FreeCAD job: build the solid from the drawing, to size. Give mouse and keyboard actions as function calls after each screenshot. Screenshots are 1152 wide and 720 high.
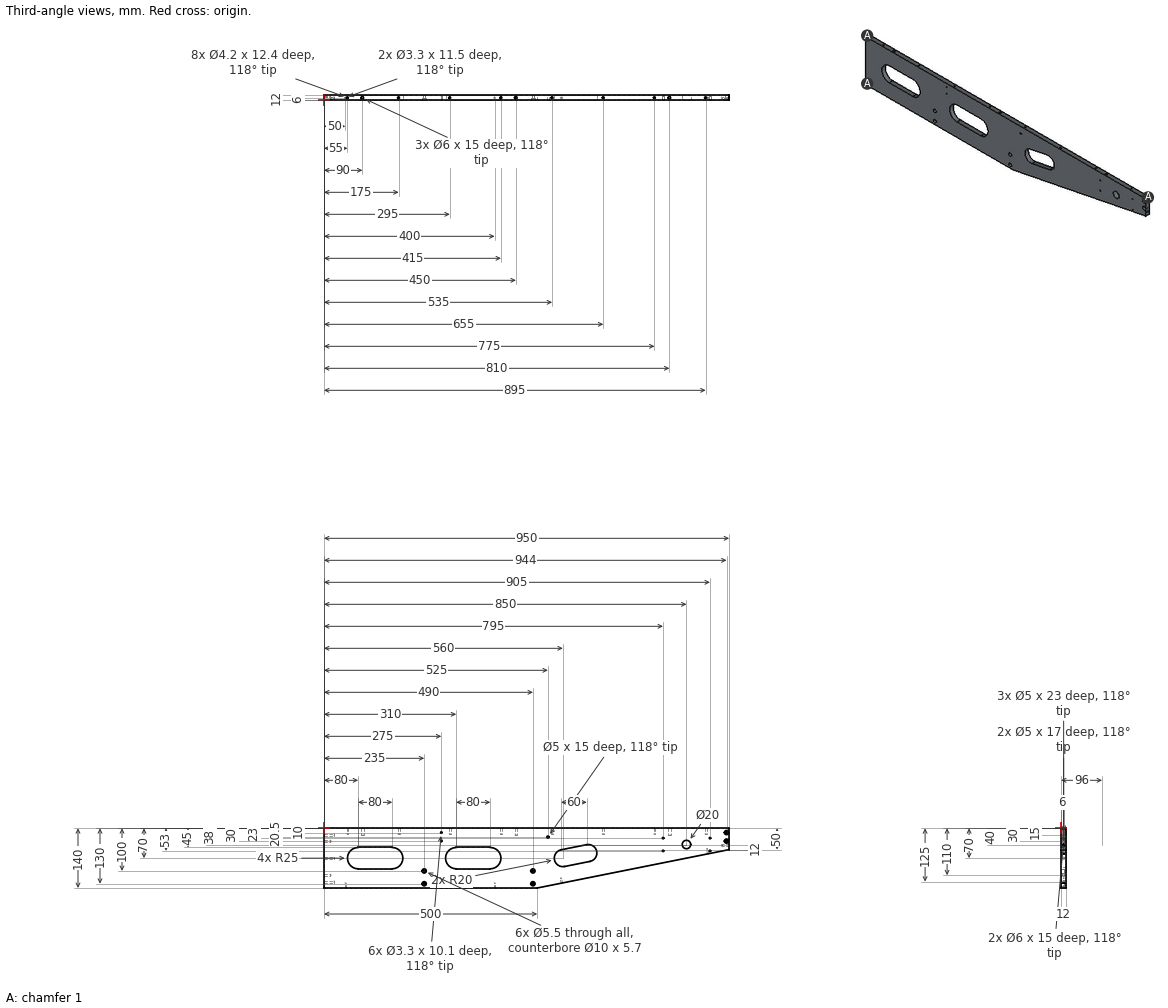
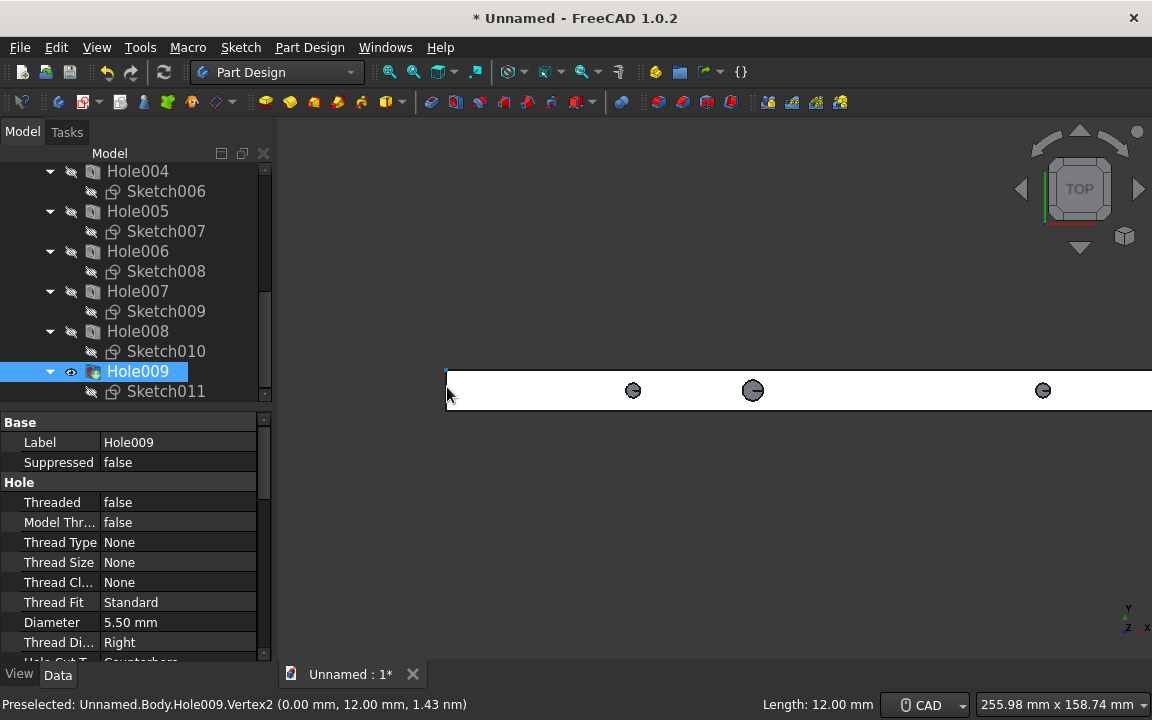
click(446, 394, ctrl)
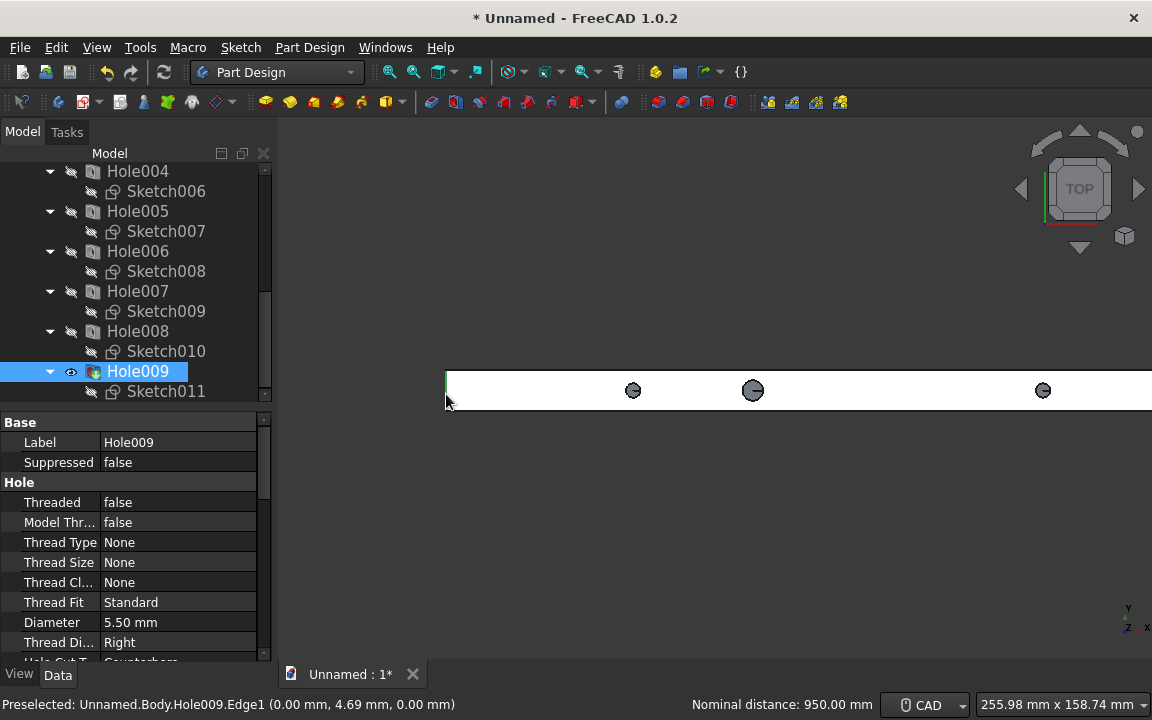
key(v)
key(f)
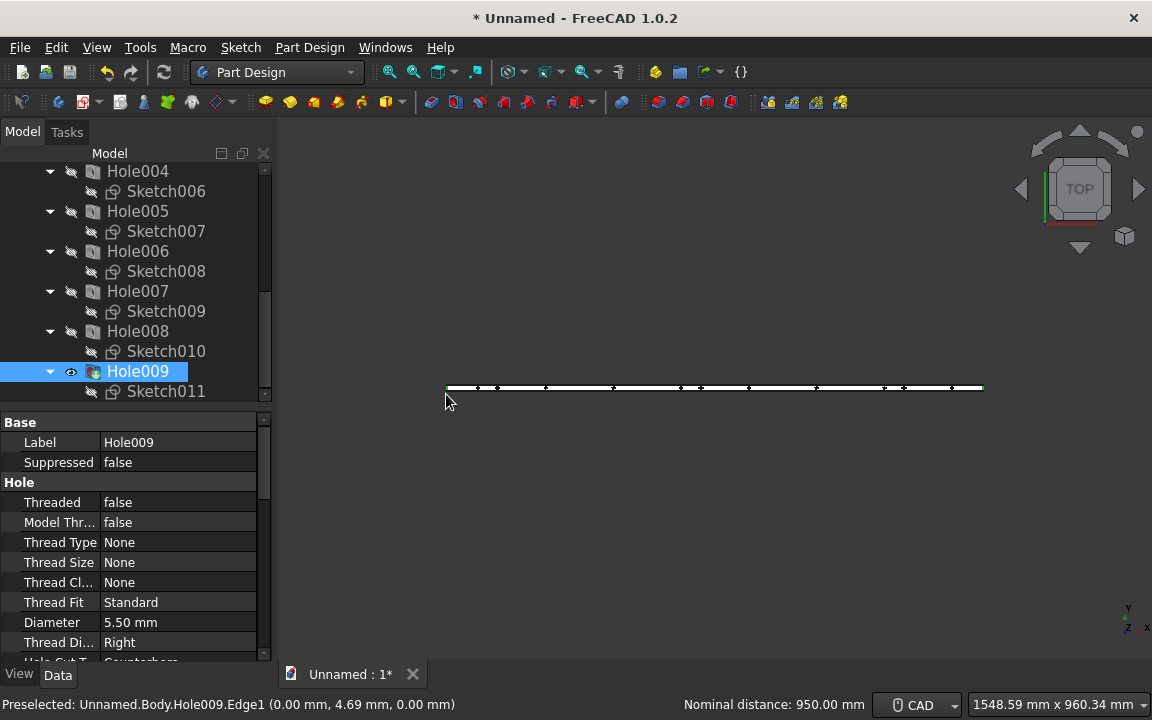
key(0)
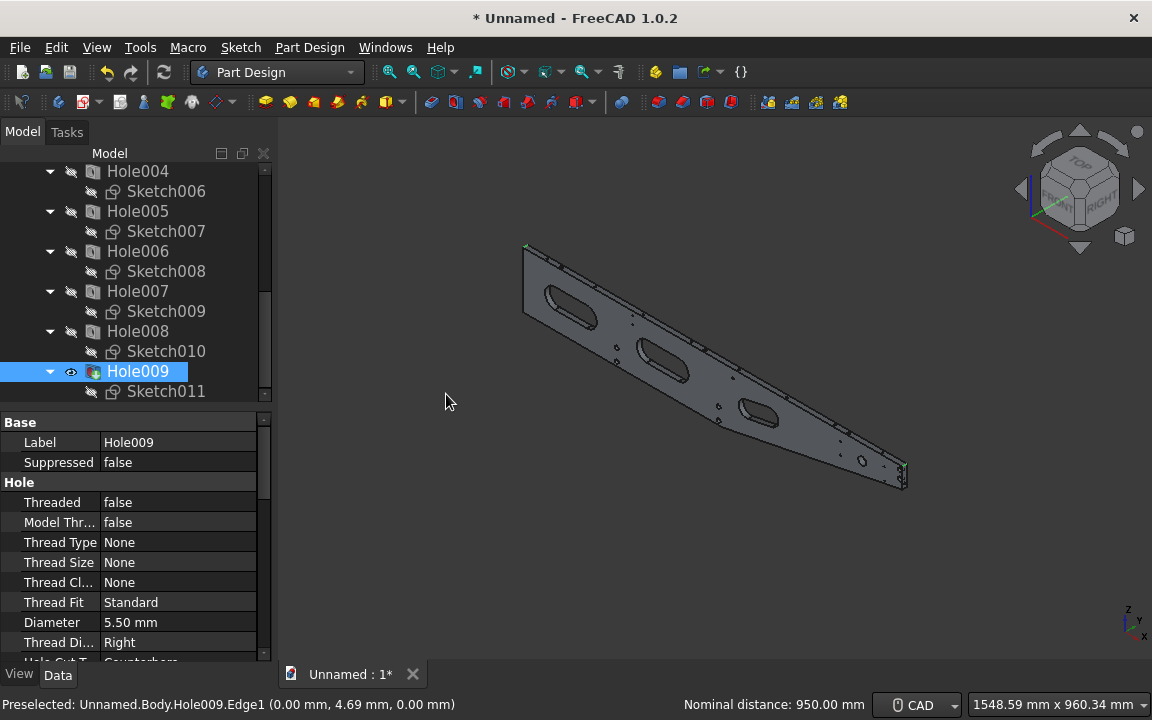
scroll(525, 310, up, 9)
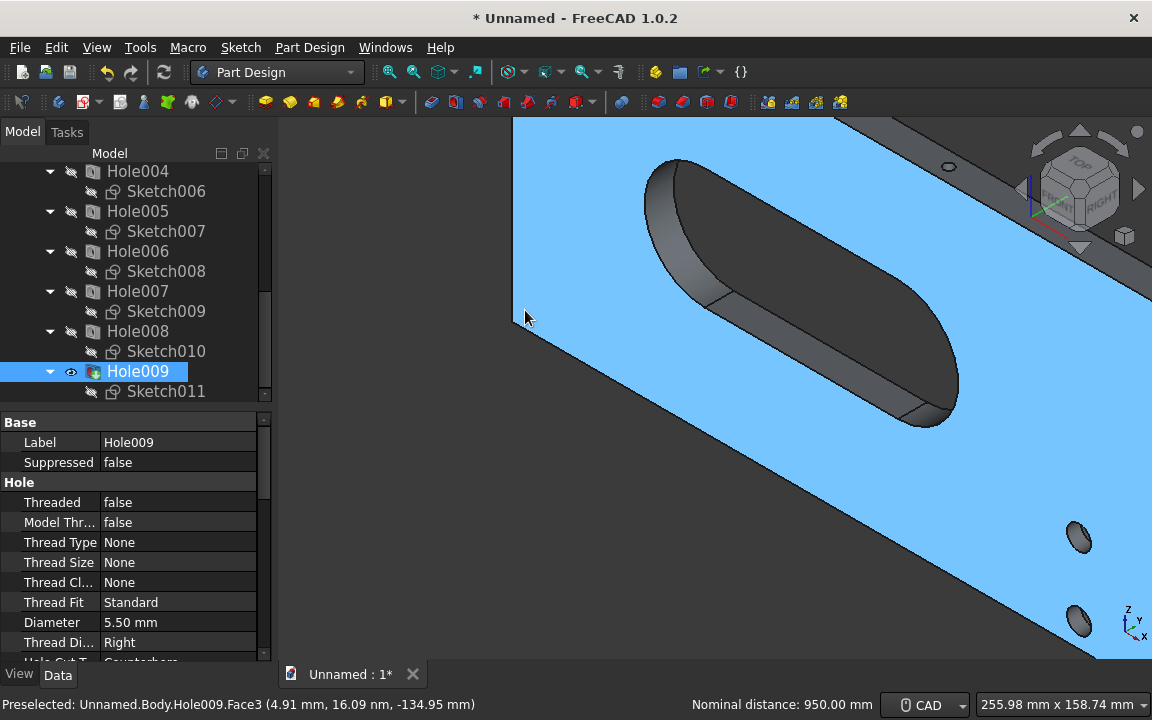
key(v)
key(f)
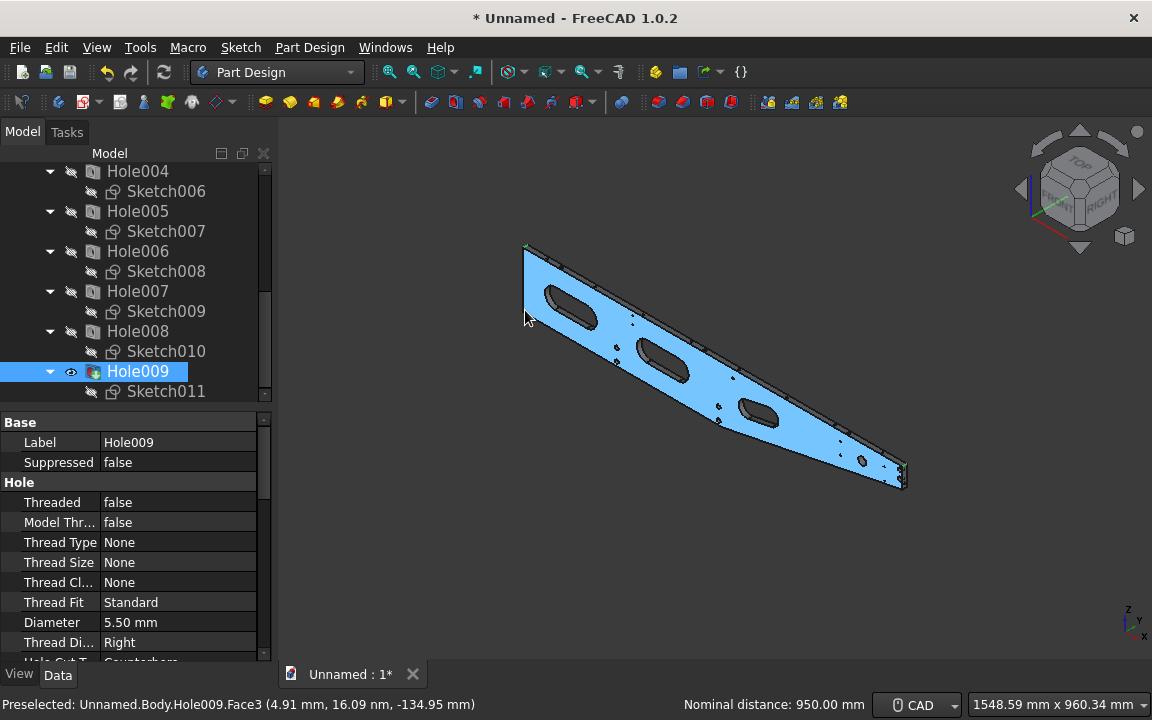
key(1)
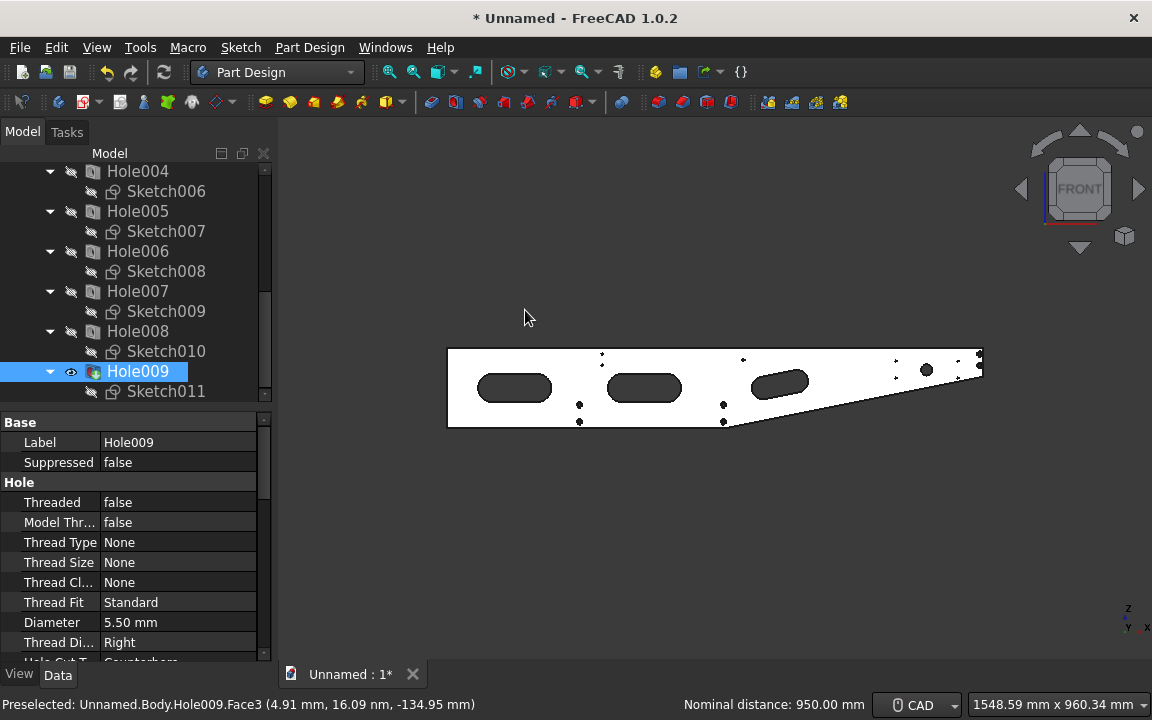
scroll(447, 427, up, 9)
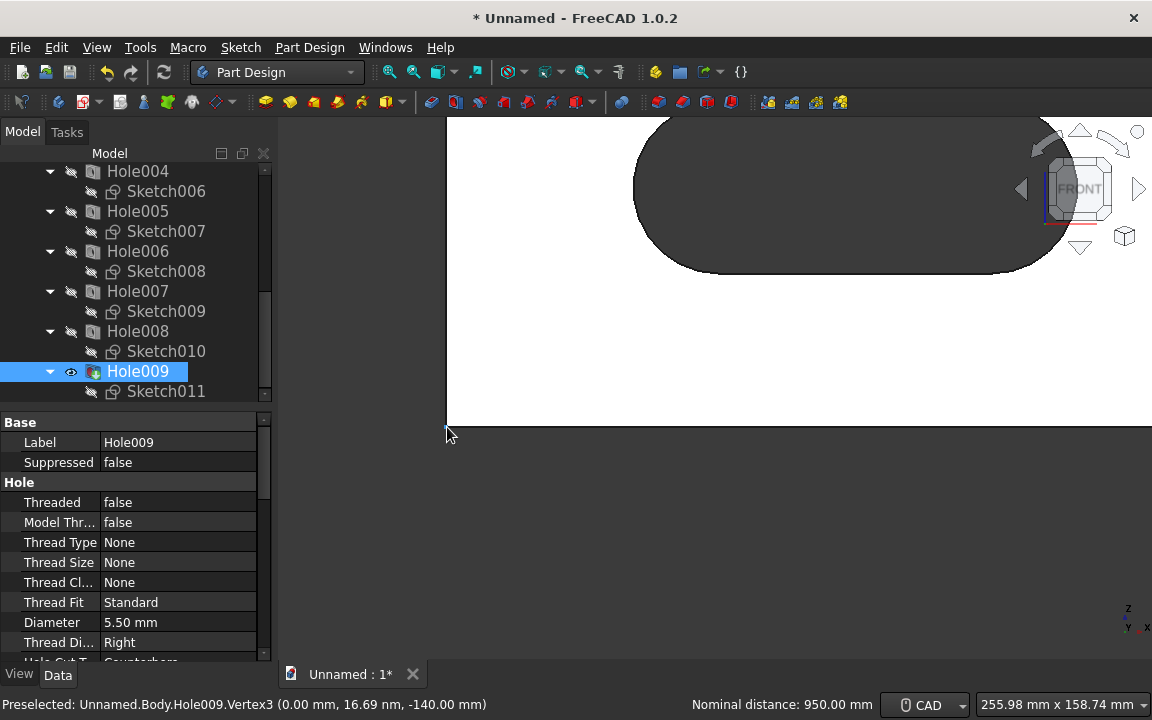
key(v)
key(f)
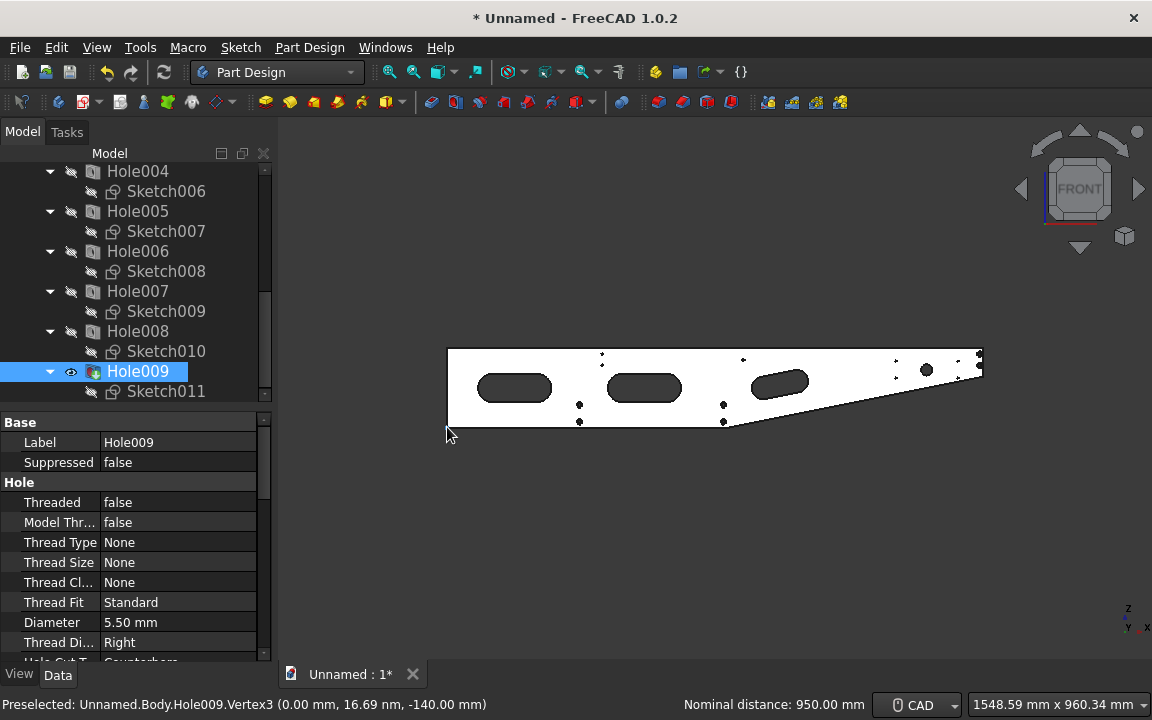
key(3)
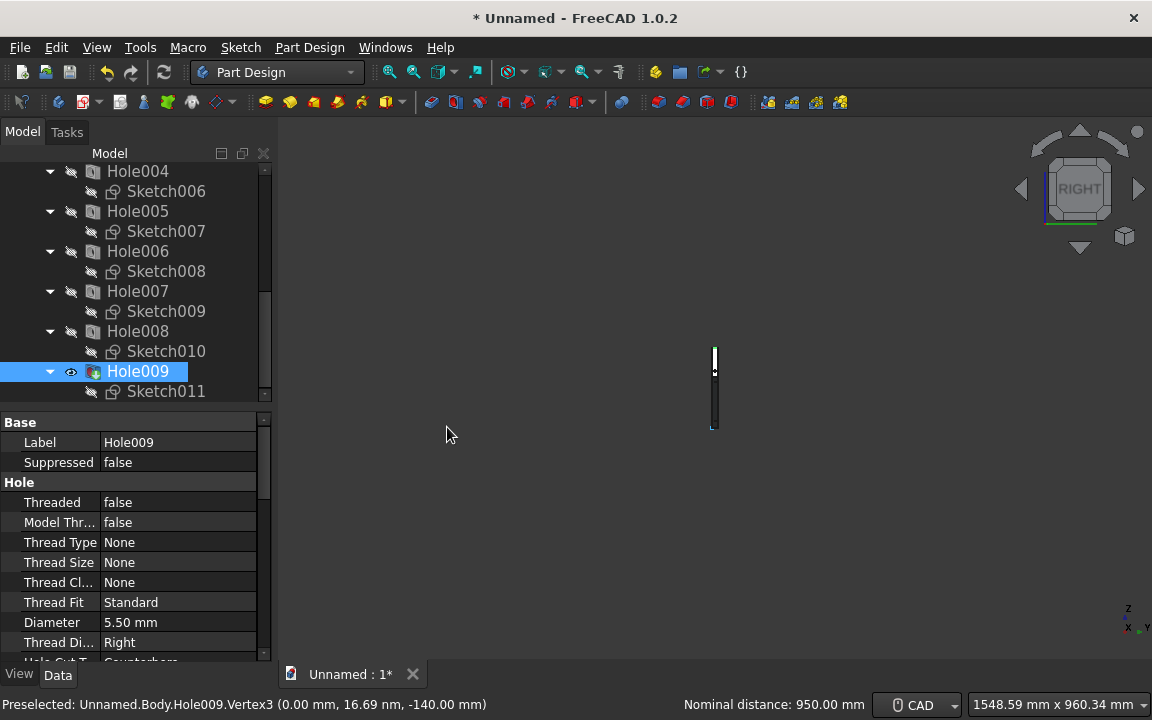
key(v)
key(f)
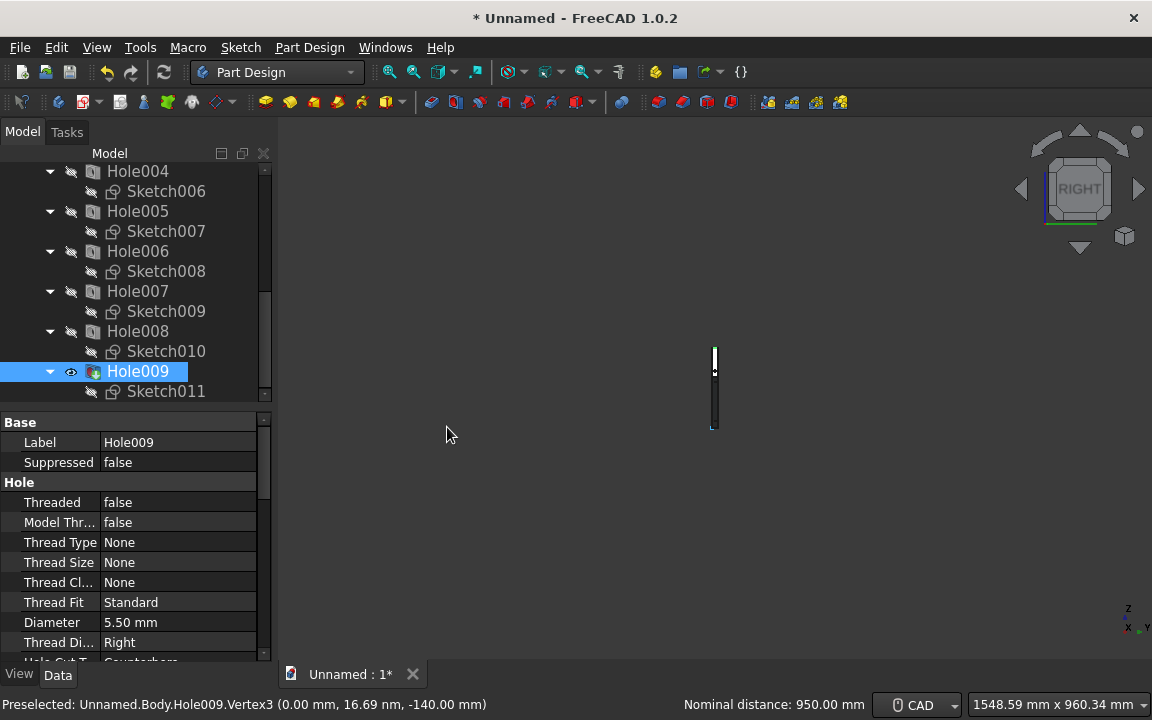
scroll(715, 427, up, 9)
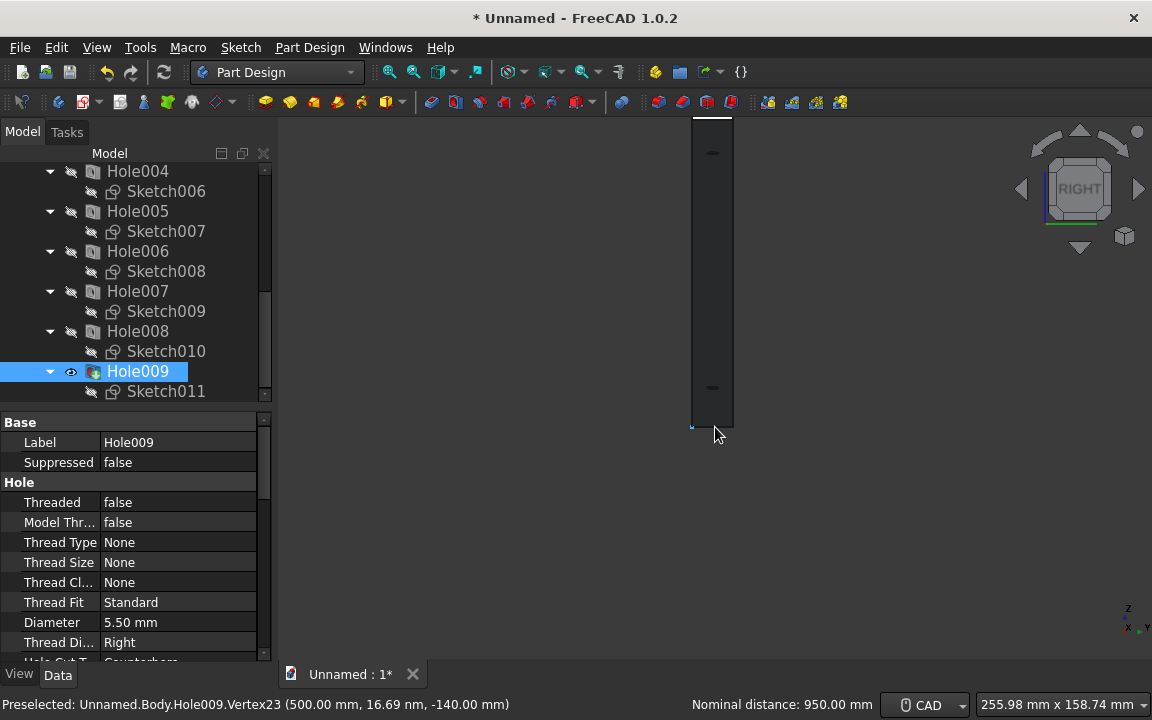
click(390, 72)